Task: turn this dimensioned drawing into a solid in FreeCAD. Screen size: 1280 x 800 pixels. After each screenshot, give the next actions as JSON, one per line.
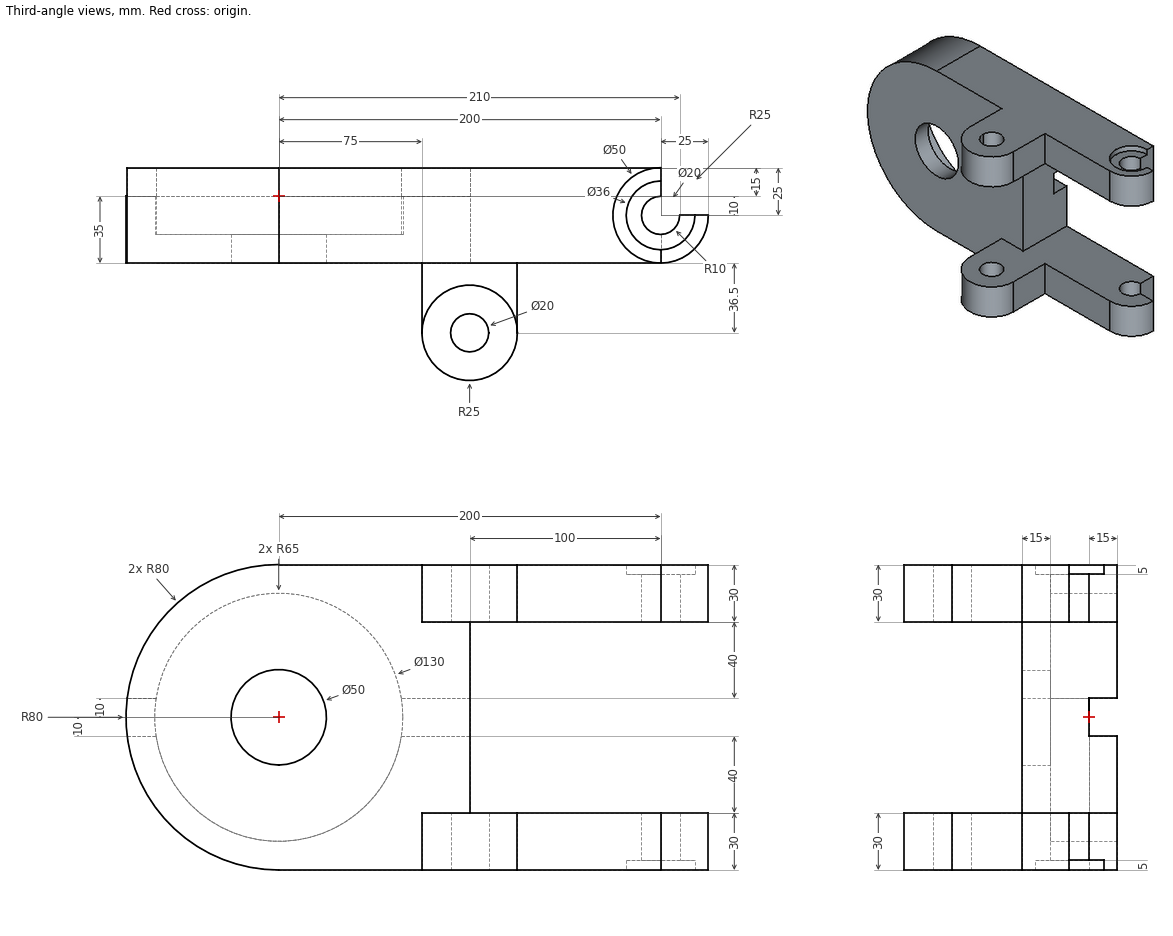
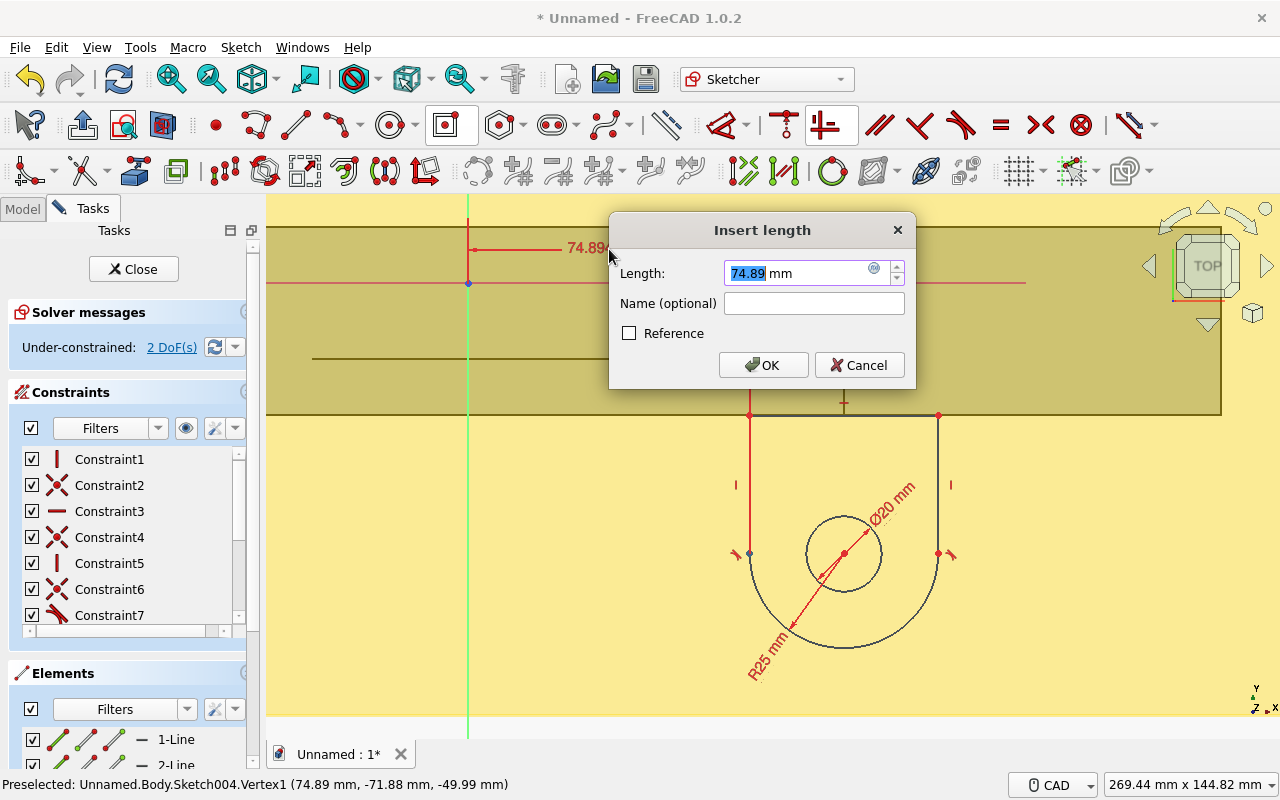
{"action": "type", "text": "75"}
{"action": "key", "text": "Return"}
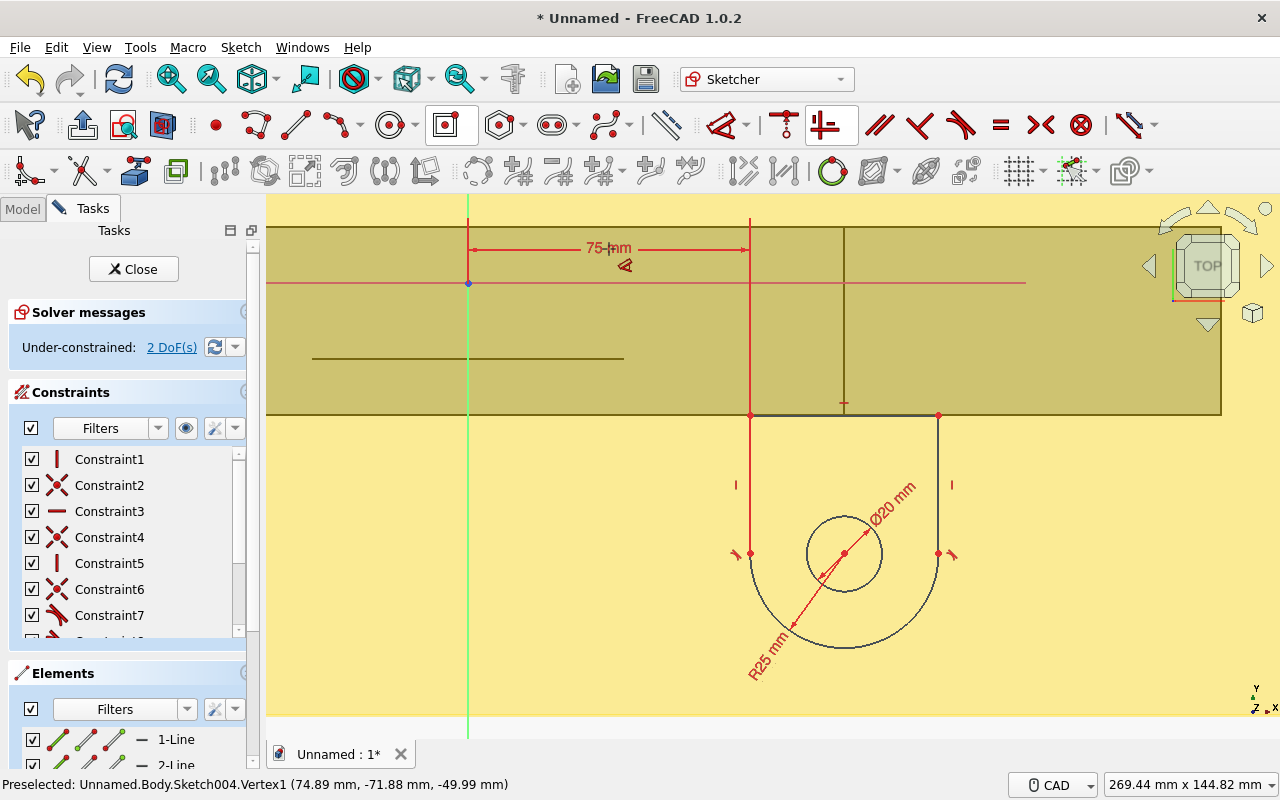
{"action": "left_click", "coordinate": [750, 416]}
{"action": "left_click", "coordinate": [434, 350]}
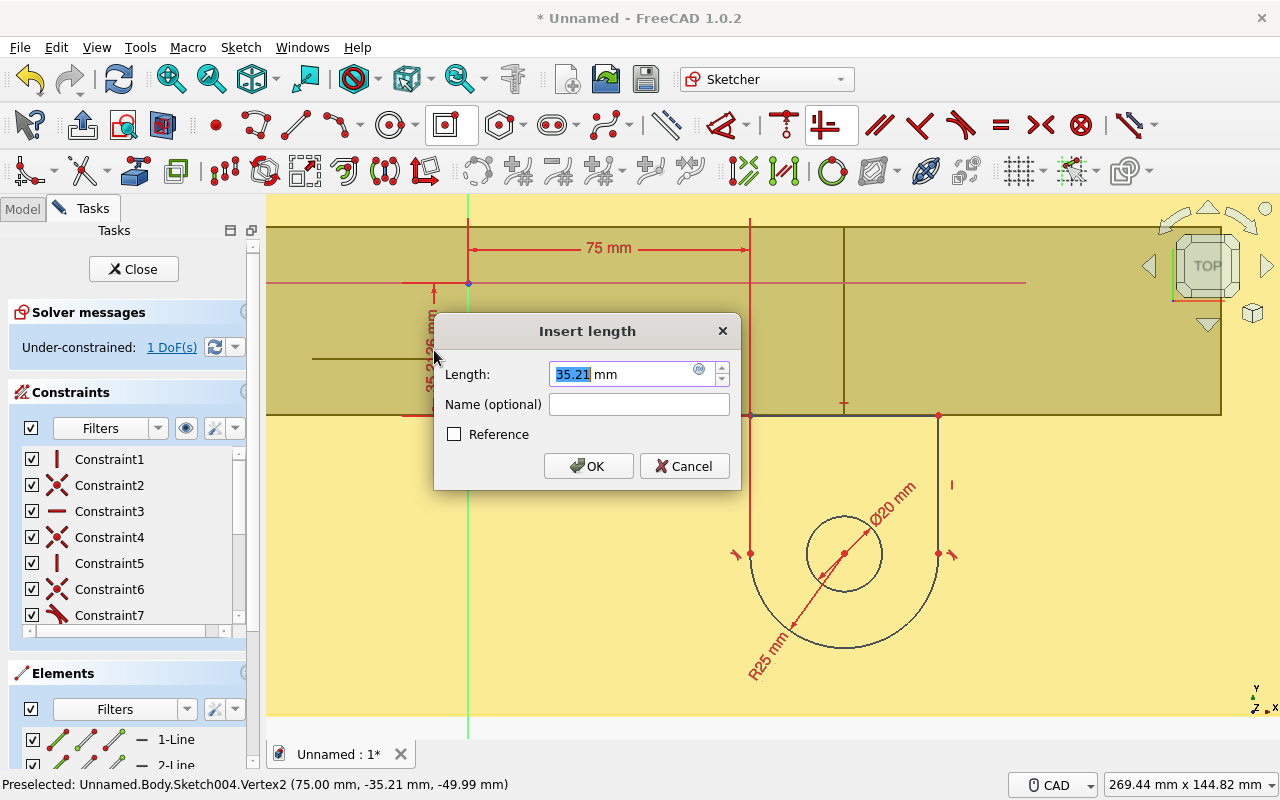
{"action": "type", "text": "35"}
{"action": "key", "text": "Return"}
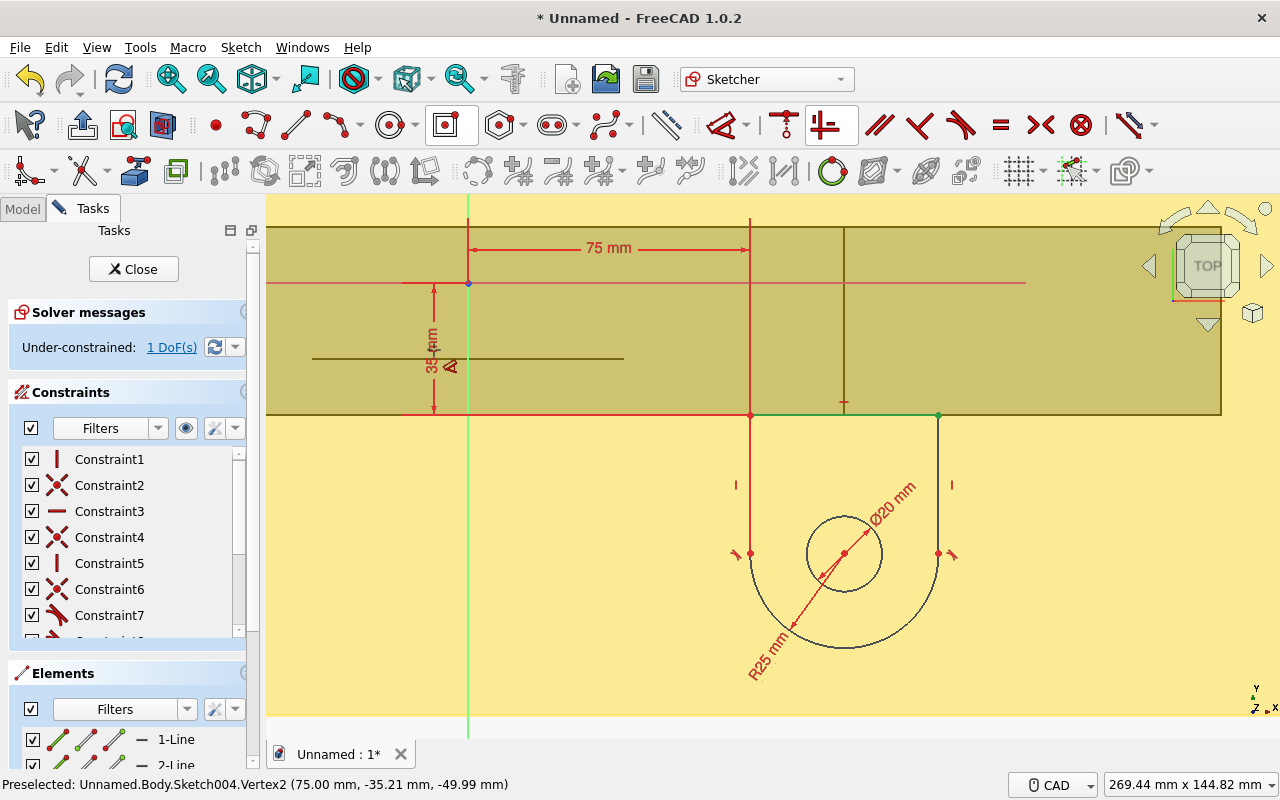
{"action": "left_click", "coordinate": [750, 512]}
{"action": "left_click", "coordinate": [784, 485]}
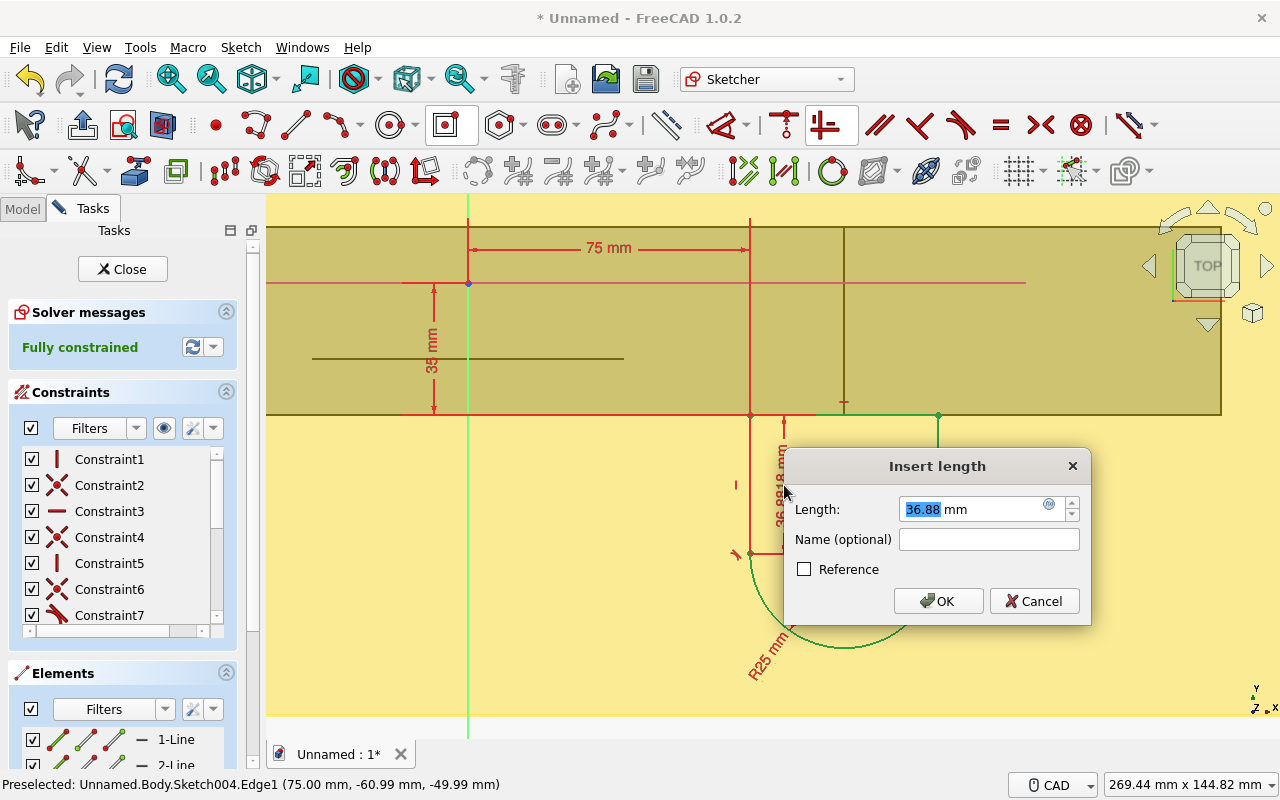
{"action": "type", "text": "36.5"}
{"action": "key", "text": "Return"}
{"action": "key", "text": "Escape"}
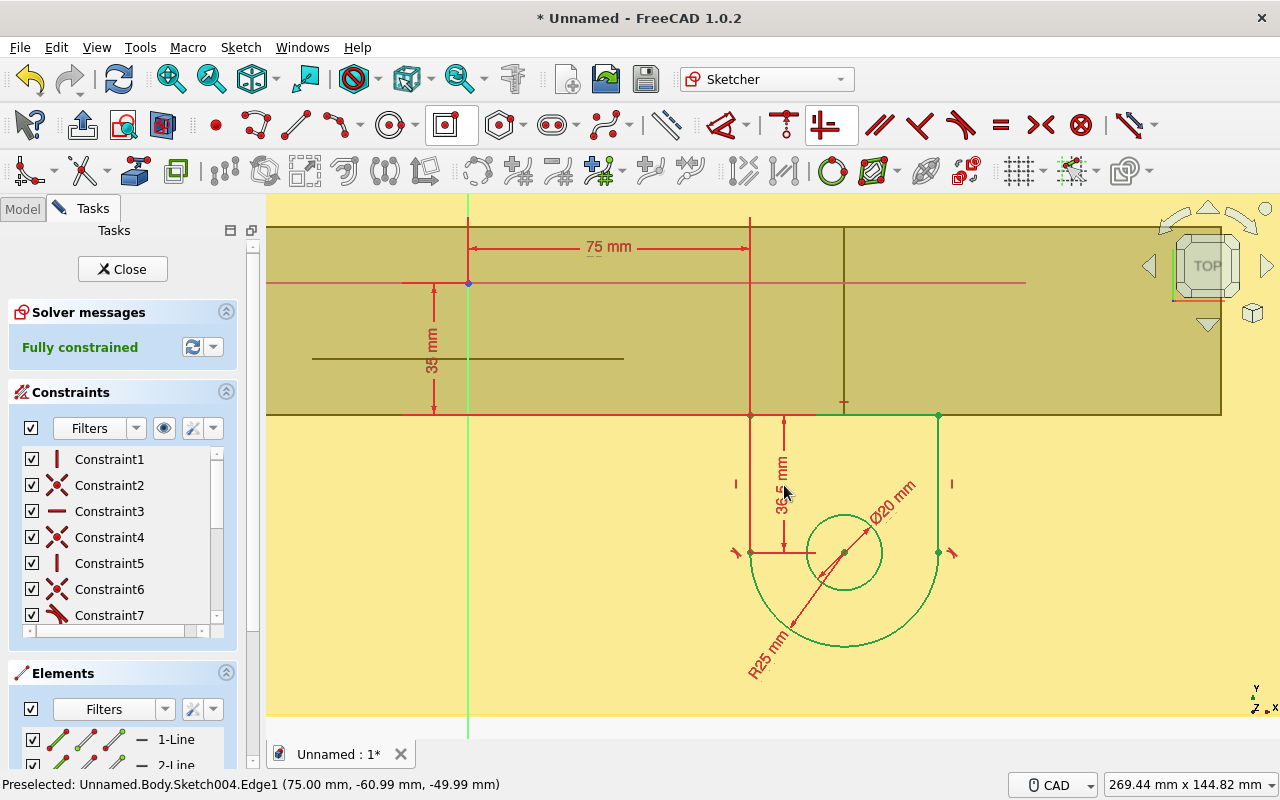
{"action": "left_click", "coordinate": [123, 269]}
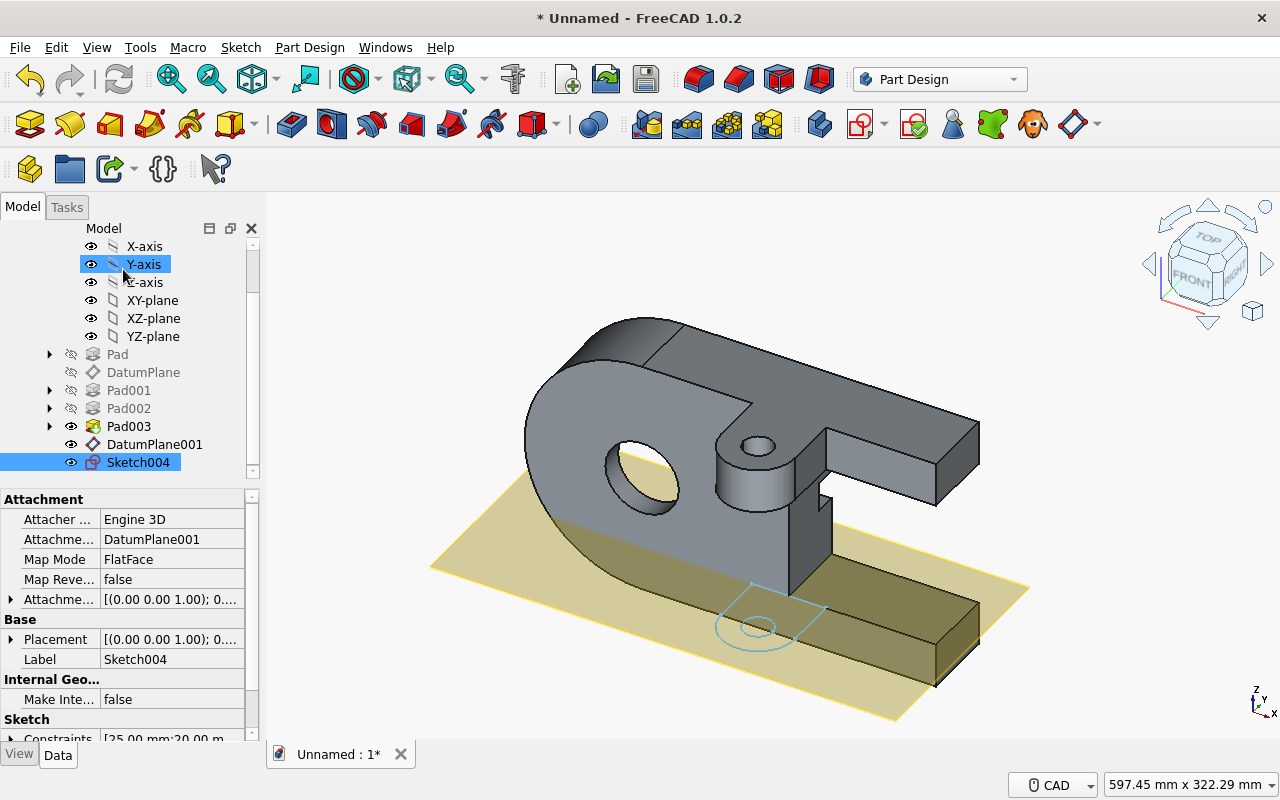
{"action": "left_click", "coordinate": [30, 124]}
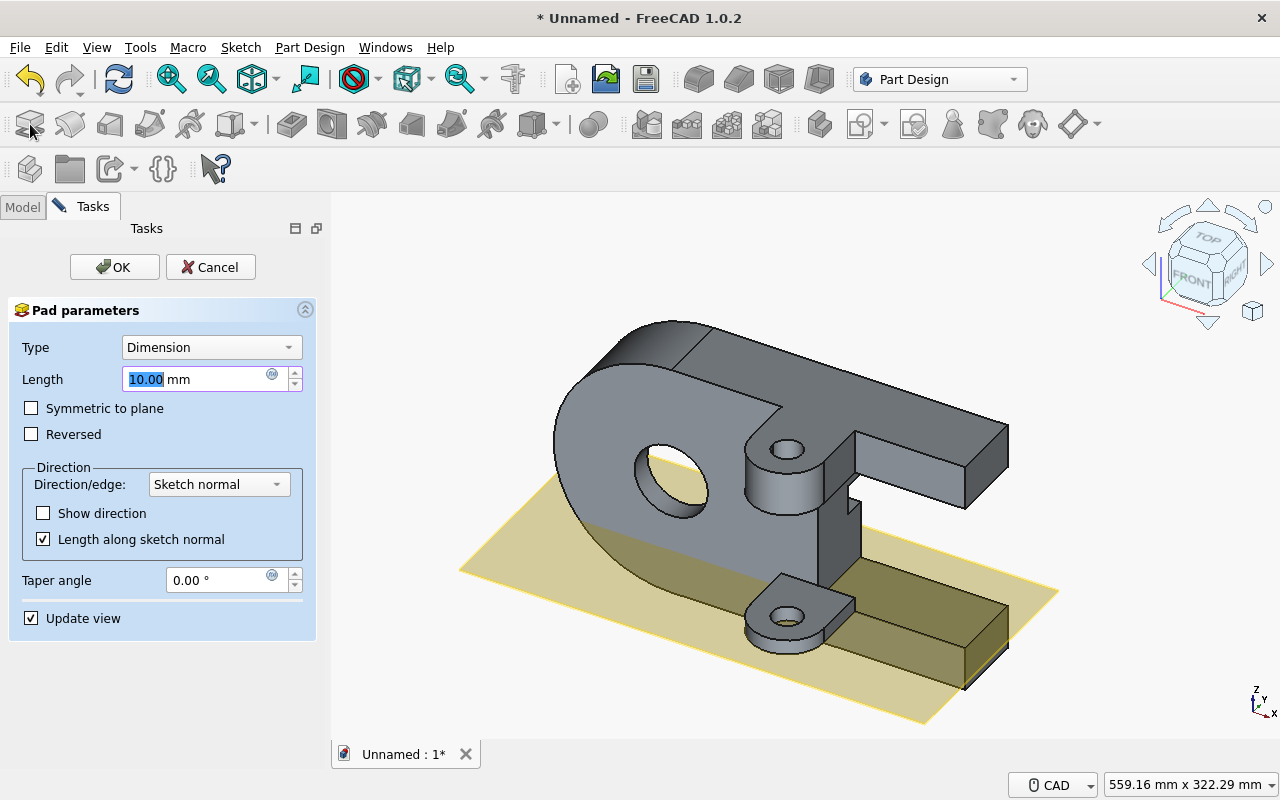
{"action": "type", "text": "30"}
{"action": "key", "text": "Tab"}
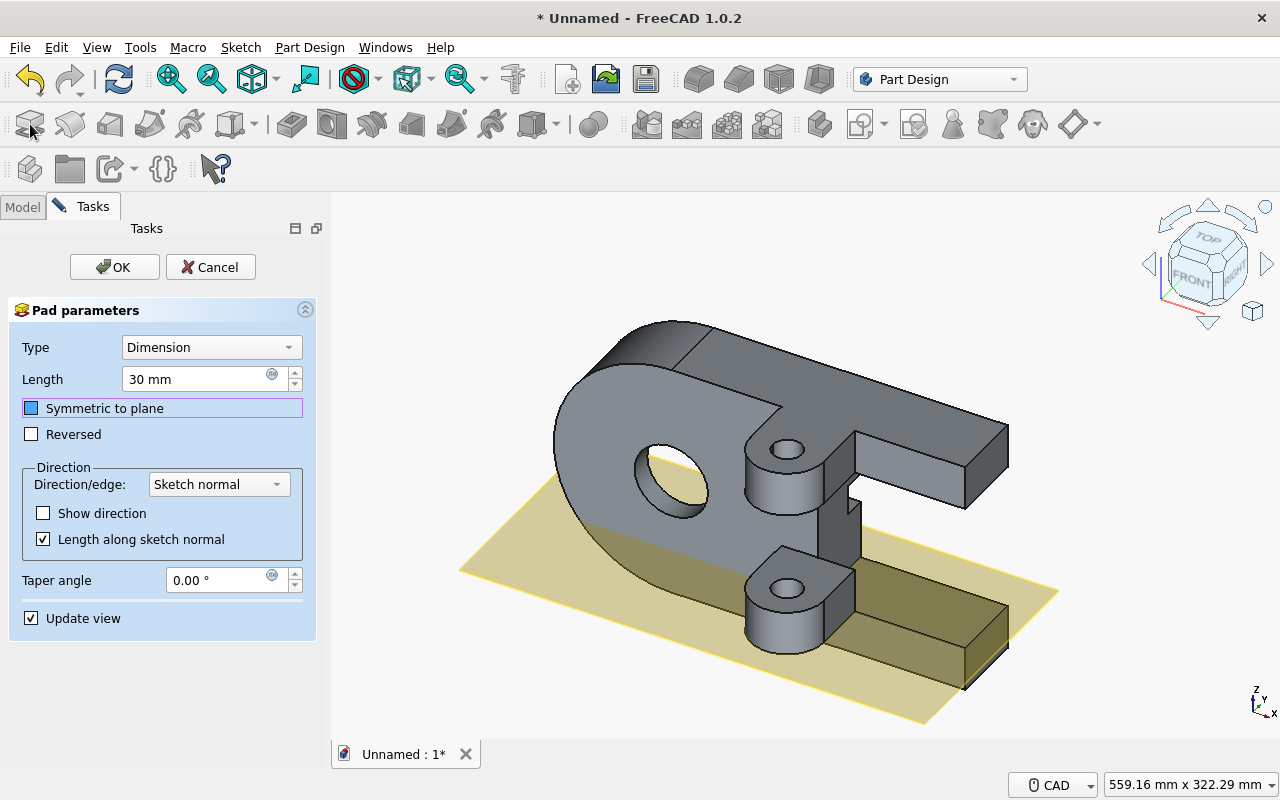
{"action": "left_click", "coordinate": [30, 434]}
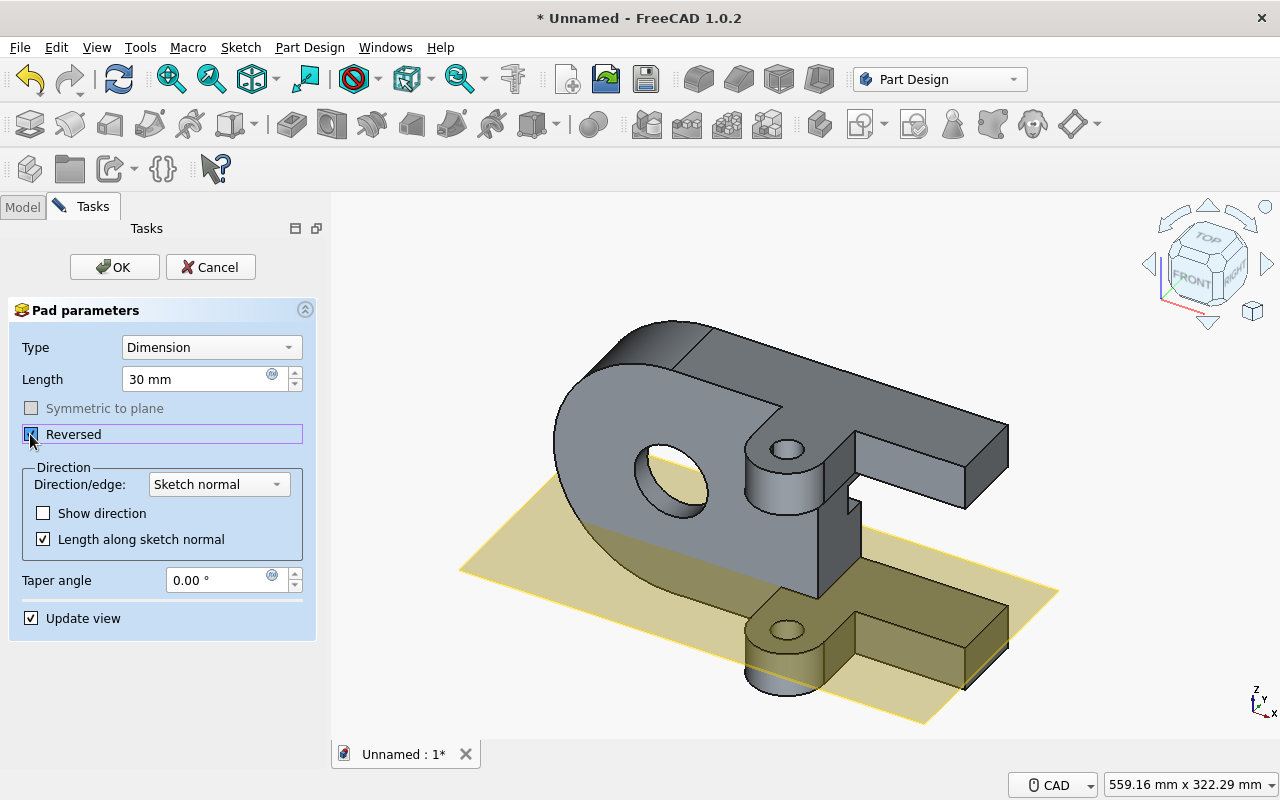
{"action": "left_click", "coordinate": [115, 267]}